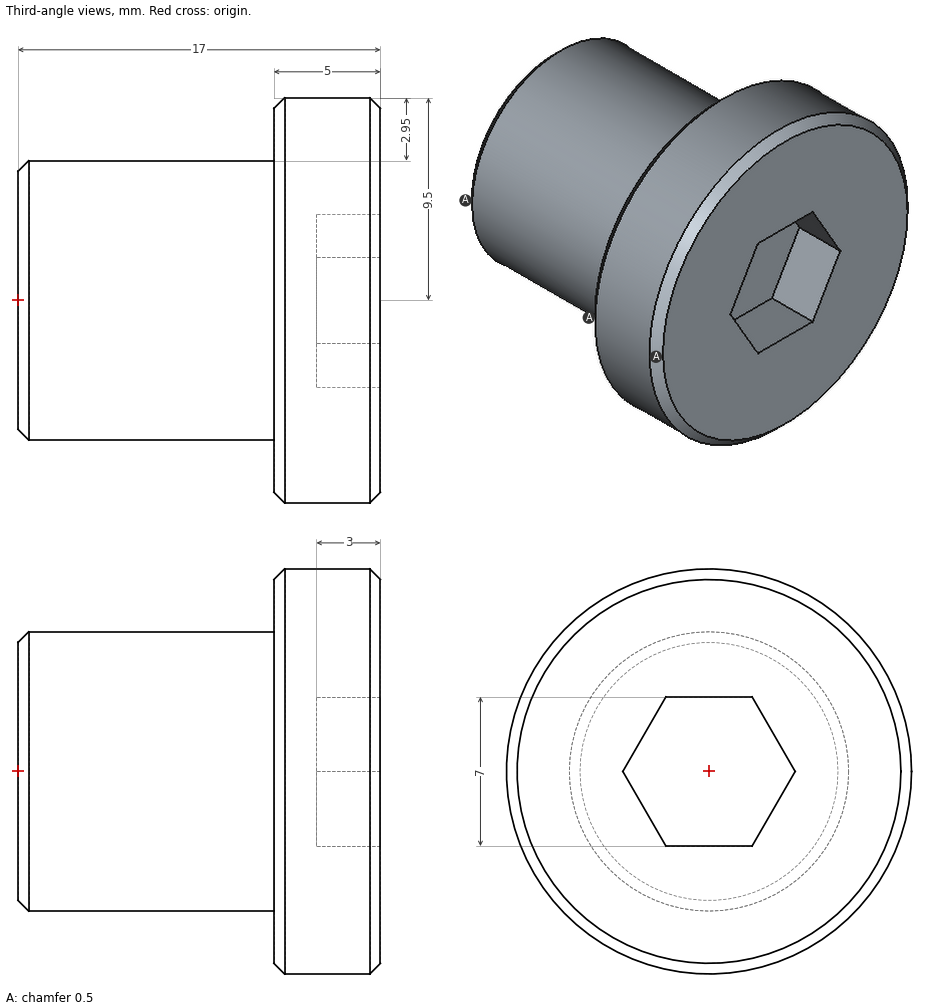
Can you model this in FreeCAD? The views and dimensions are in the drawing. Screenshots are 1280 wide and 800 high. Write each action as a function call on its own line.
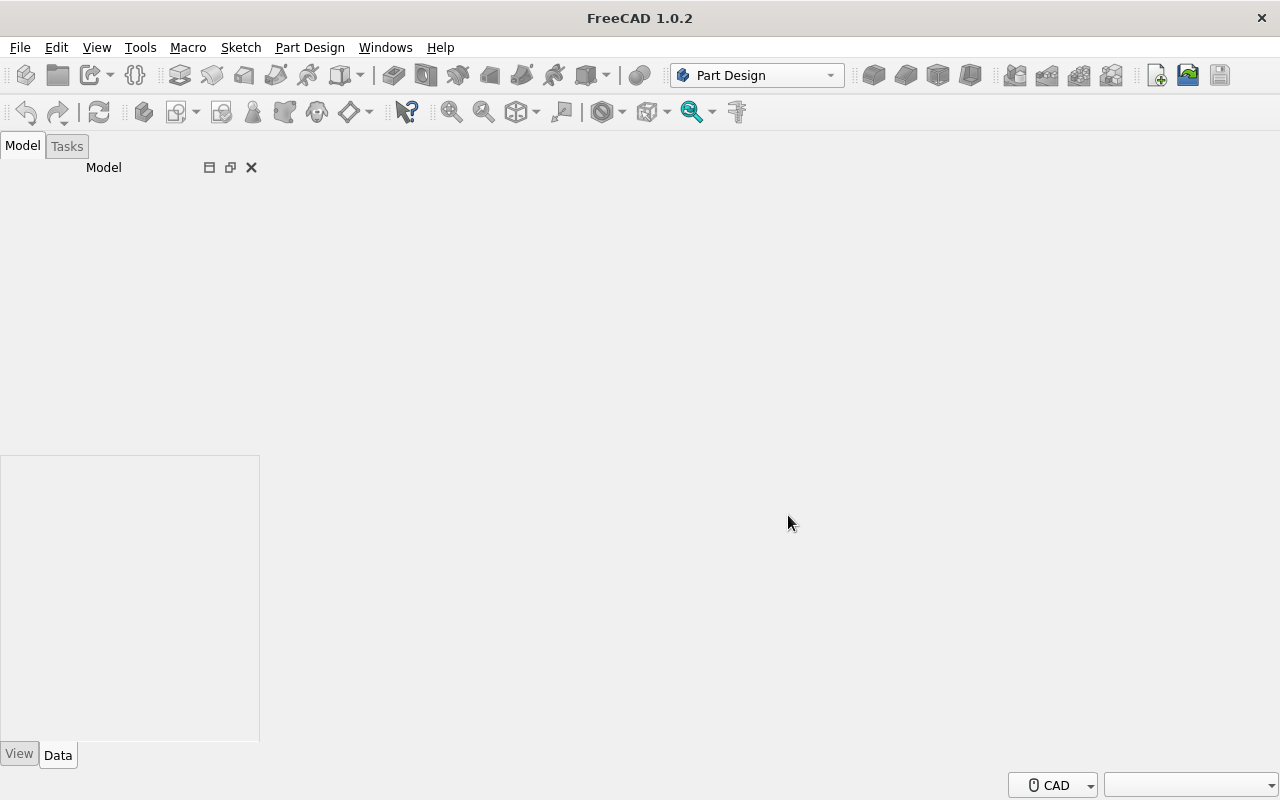
click(1156, 76)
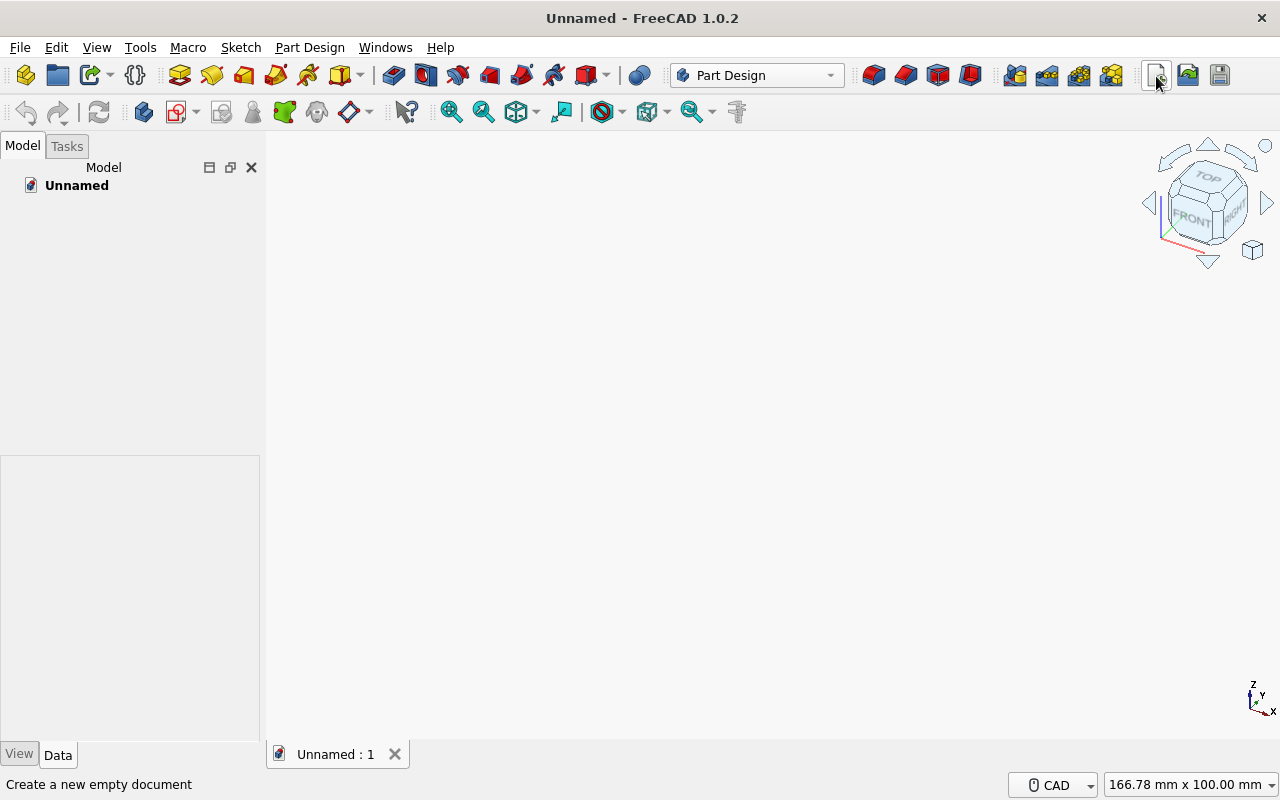
click(176, 112)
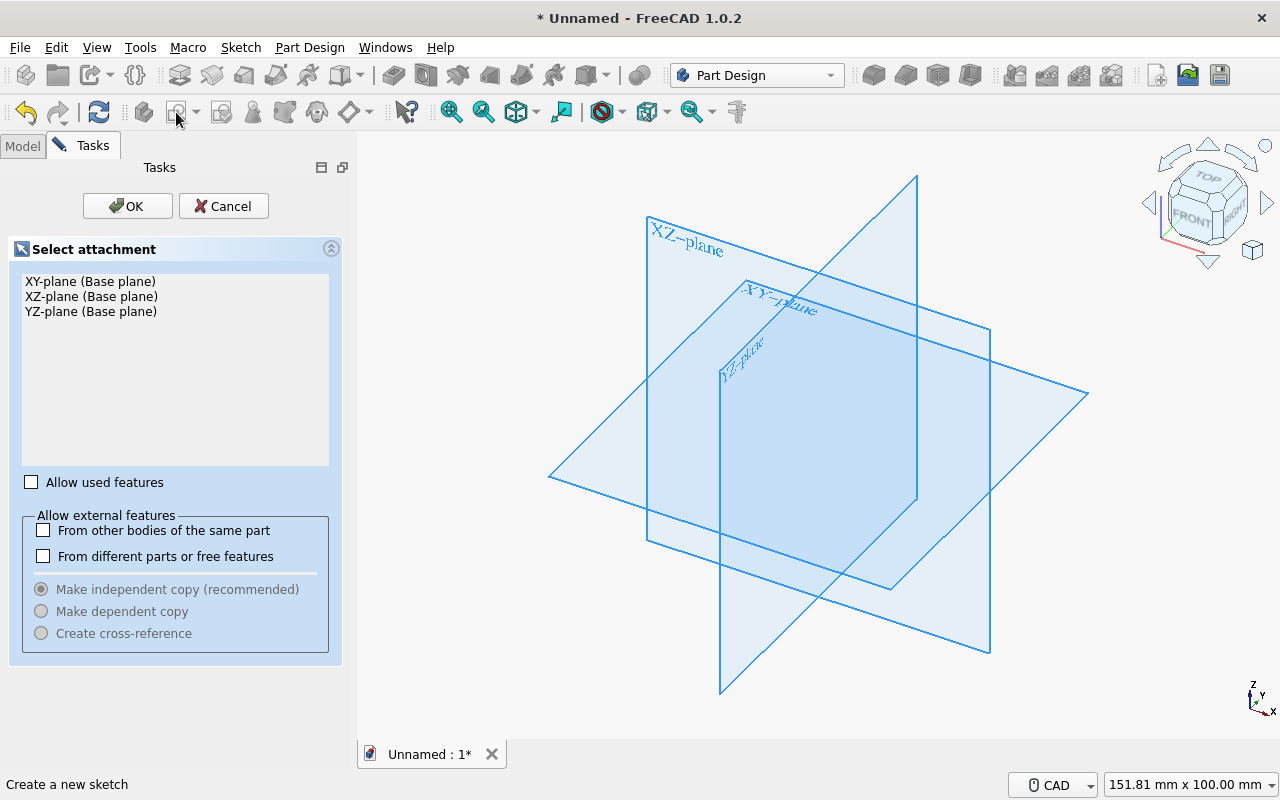
click(82, 282)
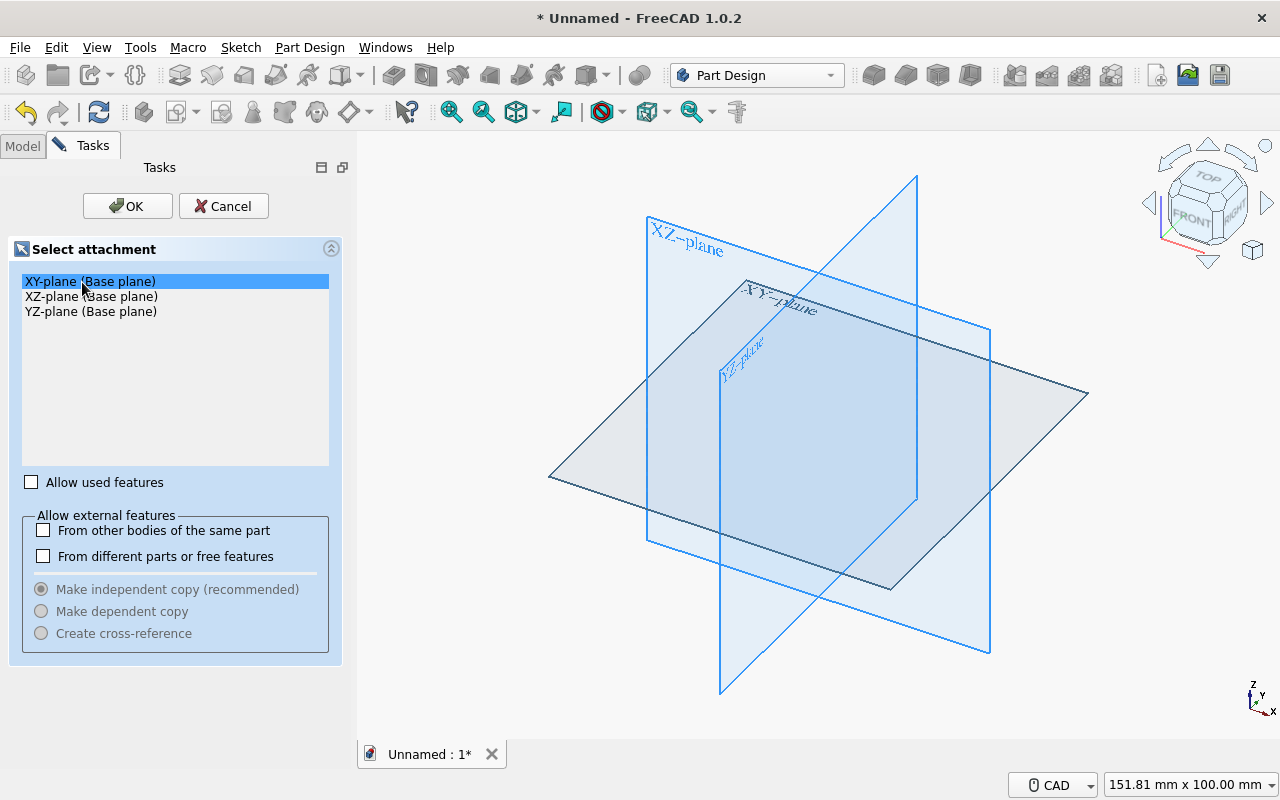
click(128, 206)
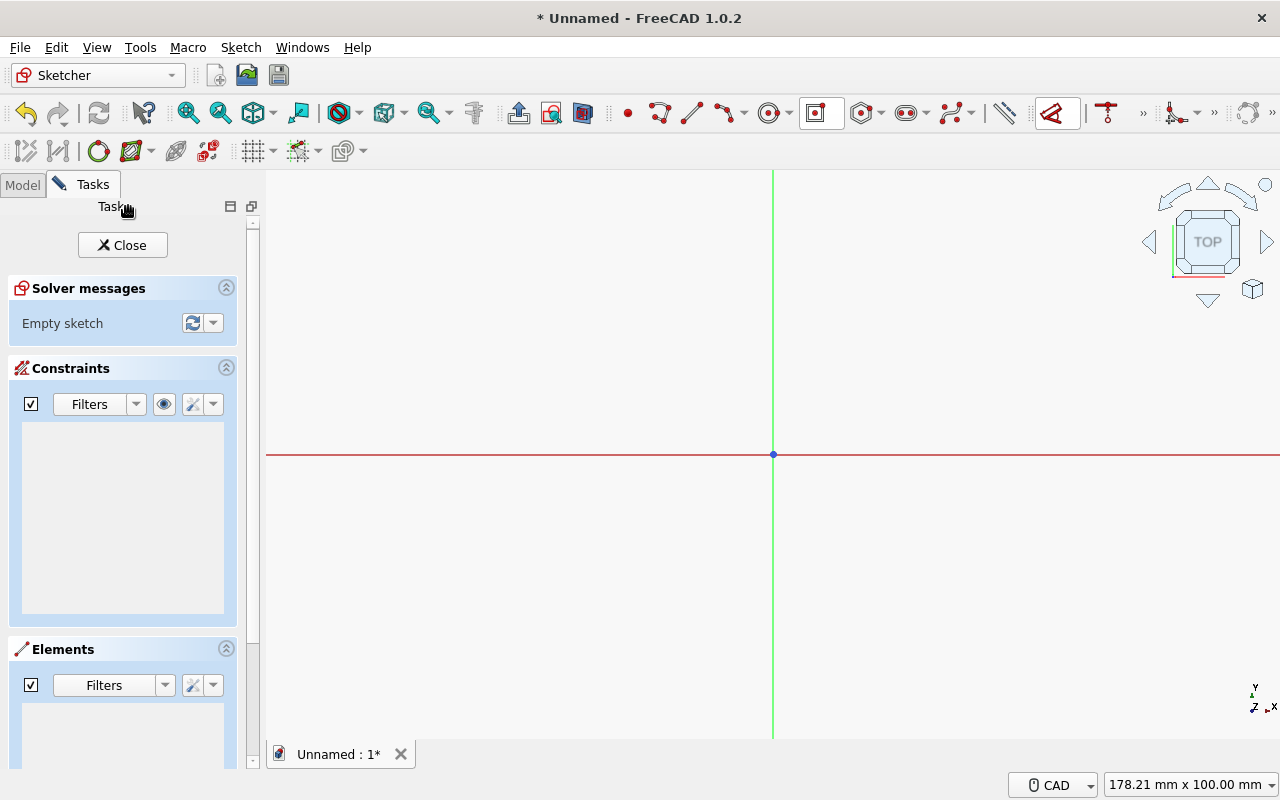
scroll(845, 422, up, 9)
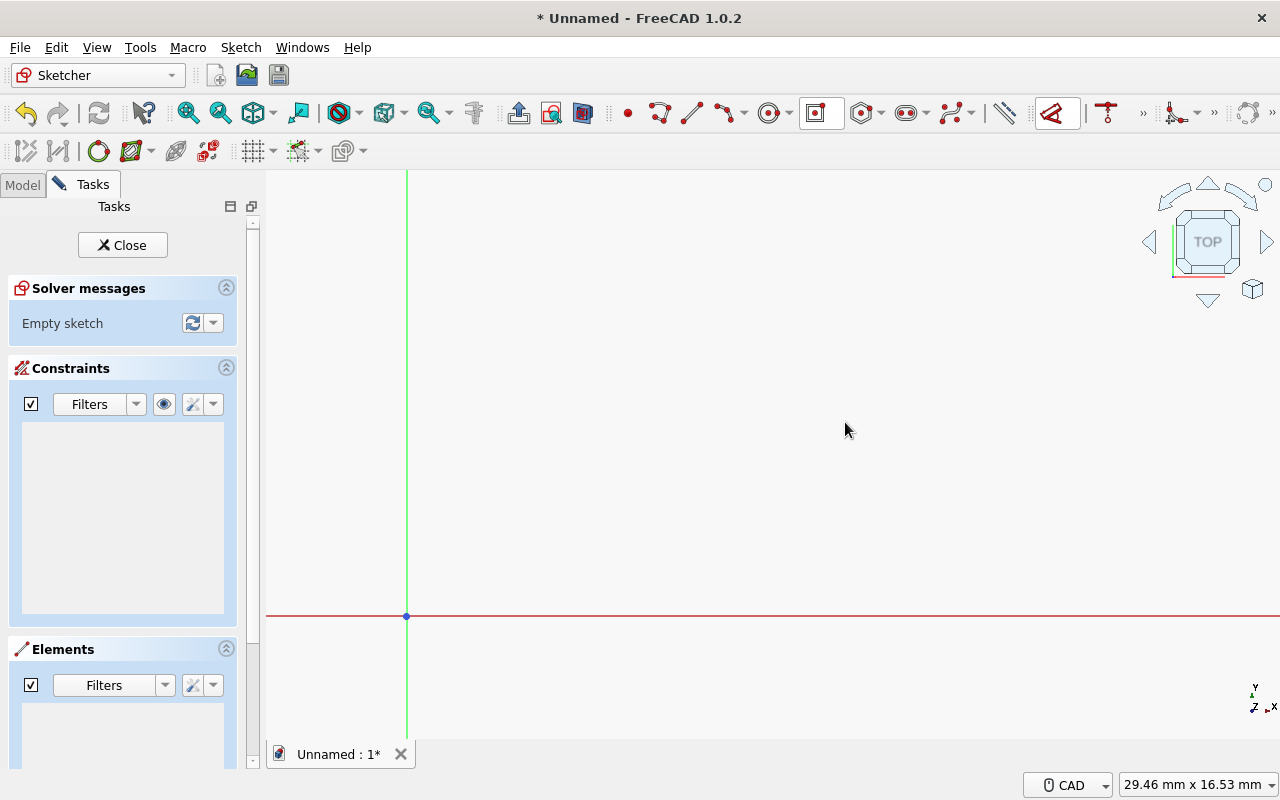
click(660, 114)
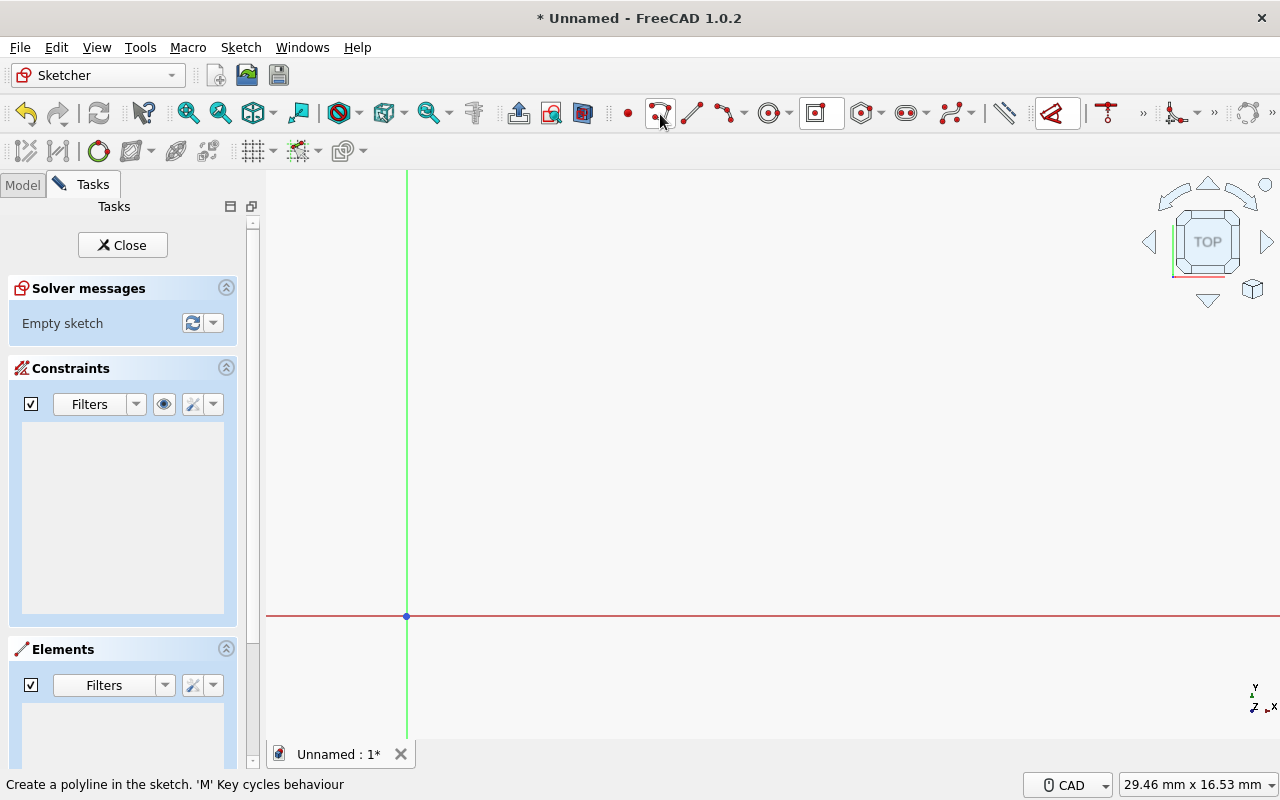
click(407, 616)
click(992, 607)
click(992, 289)
click(820, 289)
click(820, 391)
click(416, 391)
click(407, 616)
key(Escape)
key(Escape)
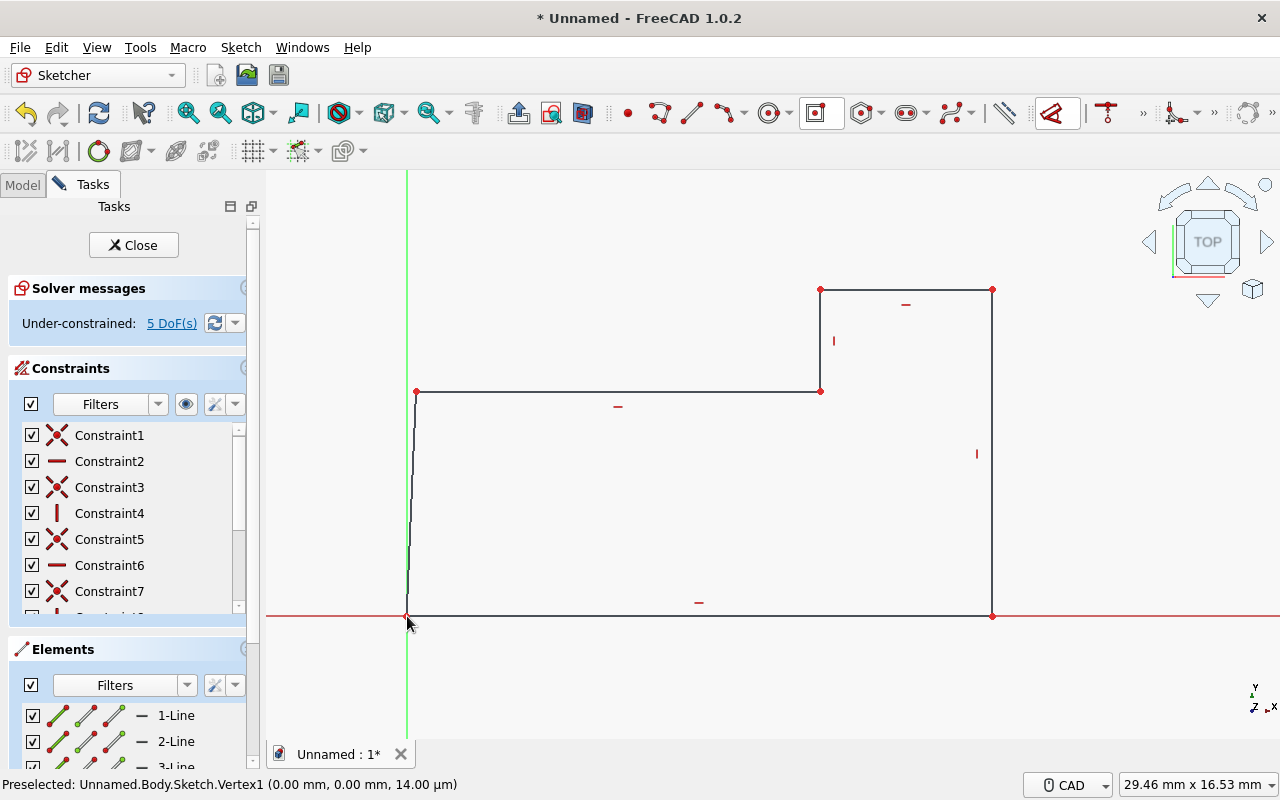
click(409, 549)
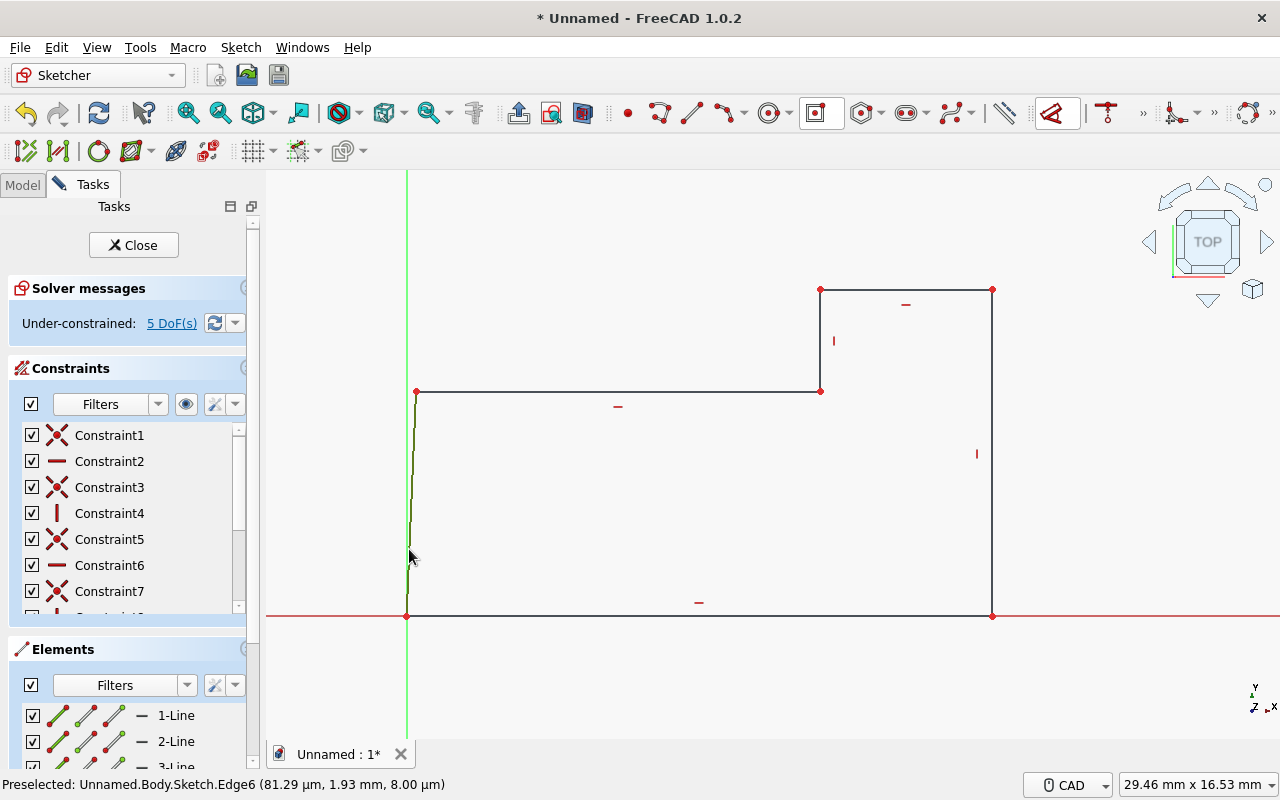
key(v)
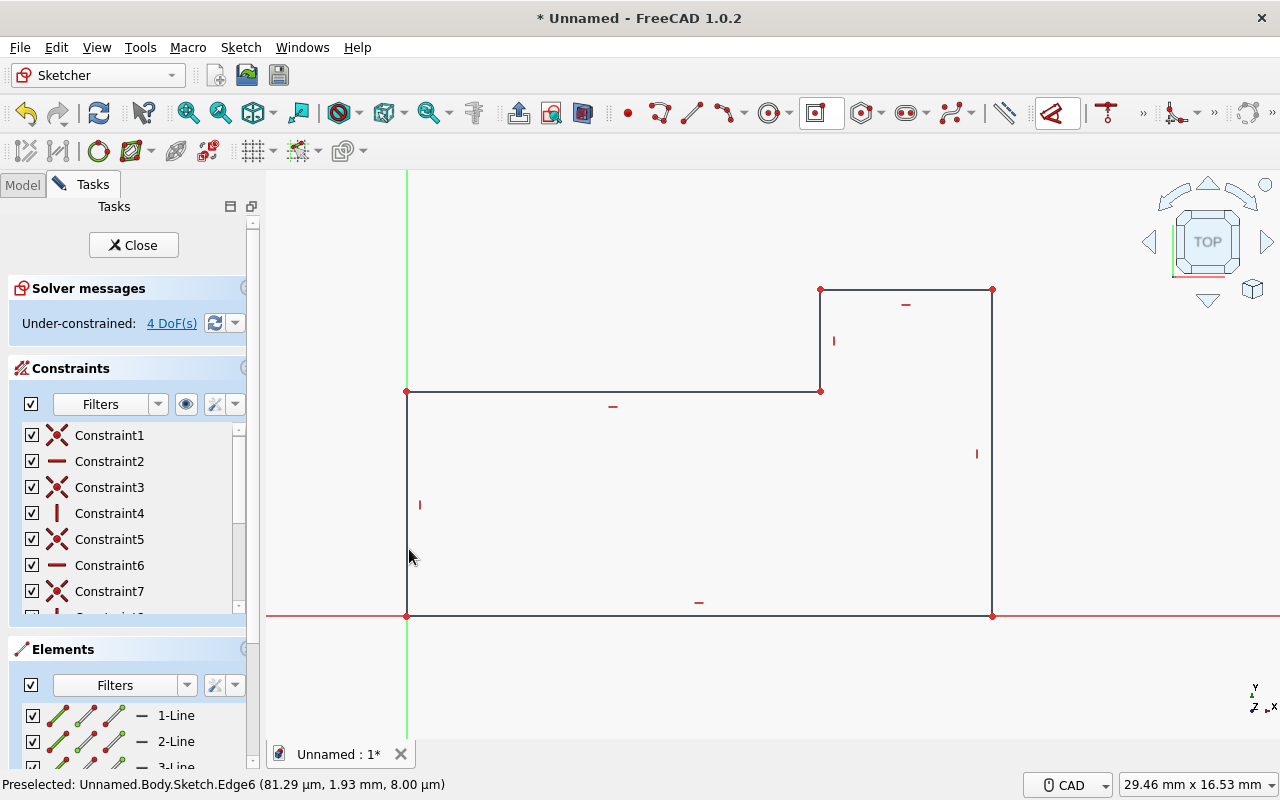
click(1052, 114)